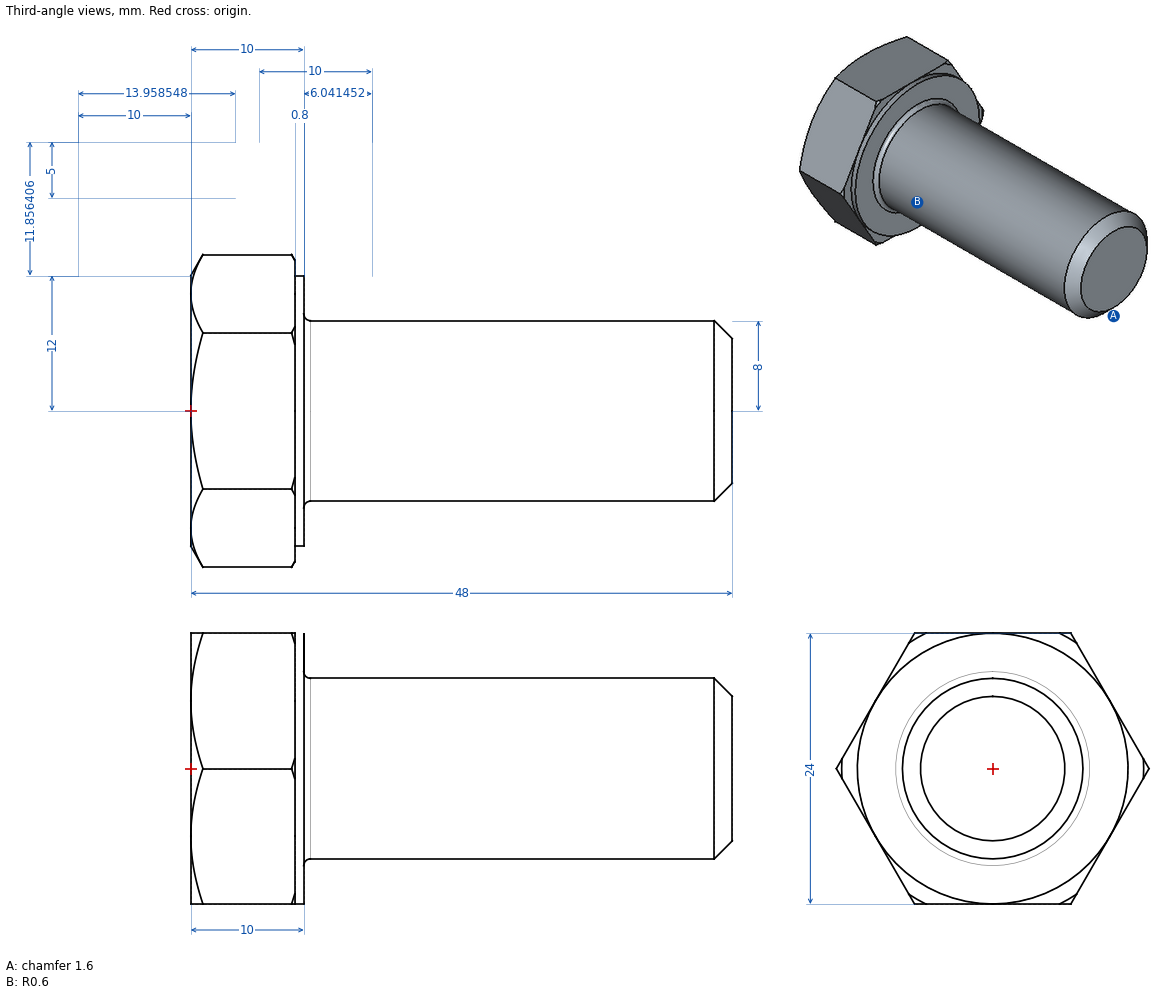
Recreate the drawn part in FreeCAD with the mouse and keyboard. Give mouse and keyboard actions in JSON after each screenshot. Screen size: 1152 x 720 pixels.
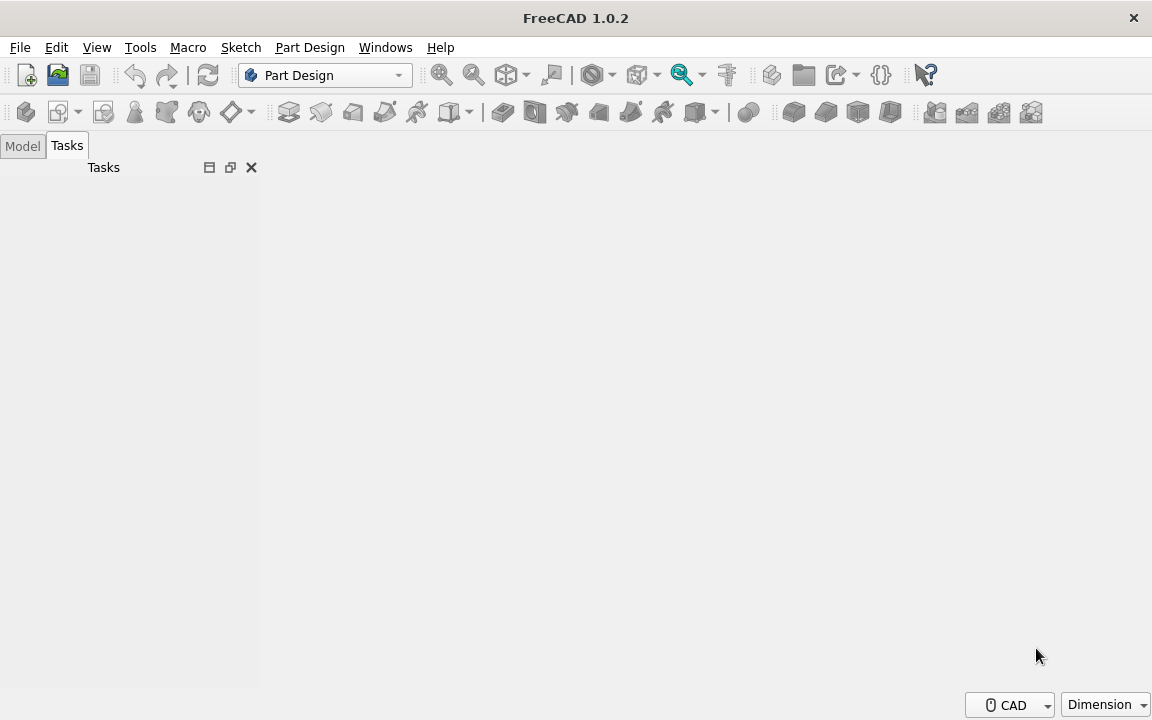
{"action": "left_click", "coordinate": [26, 76]}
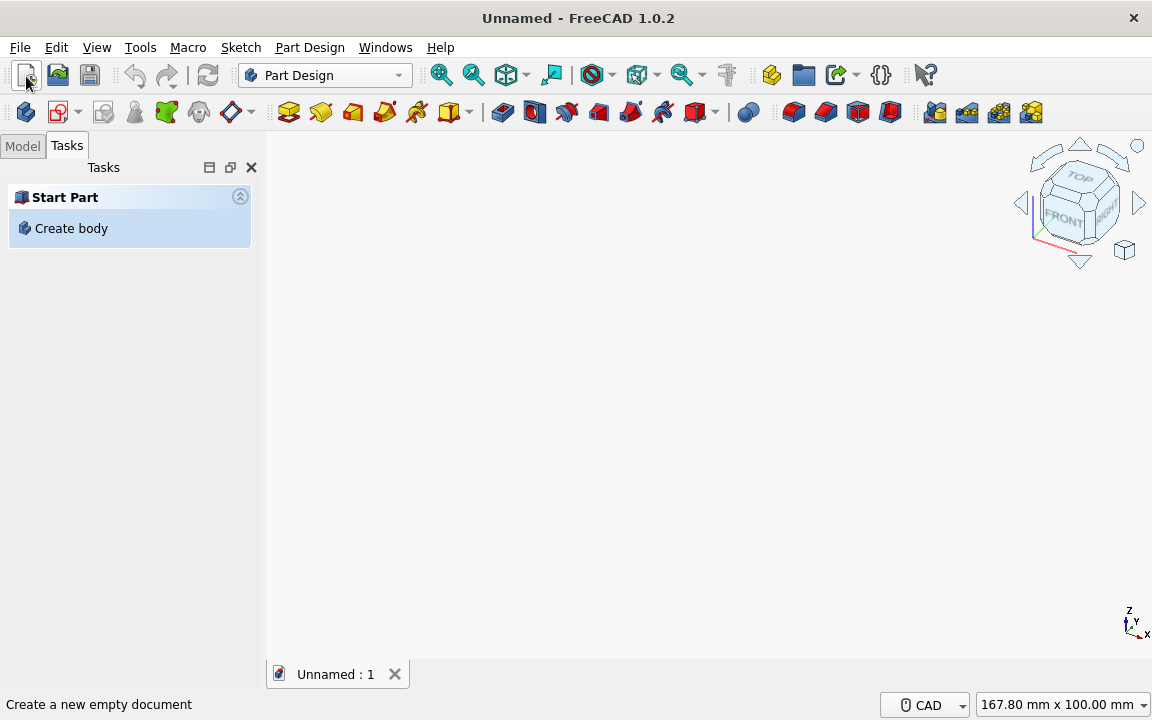
{"action": "left_click", "coordinate": [58, 112]}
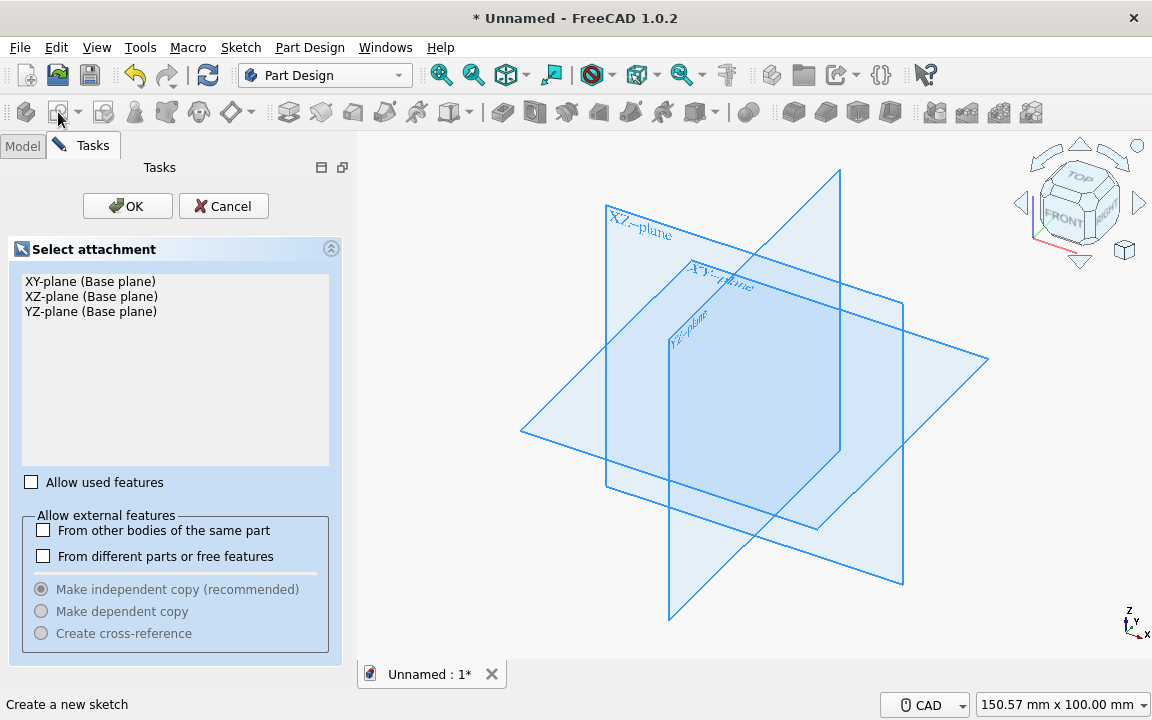
{"action": "left_click", "coordinate": [82, 312]}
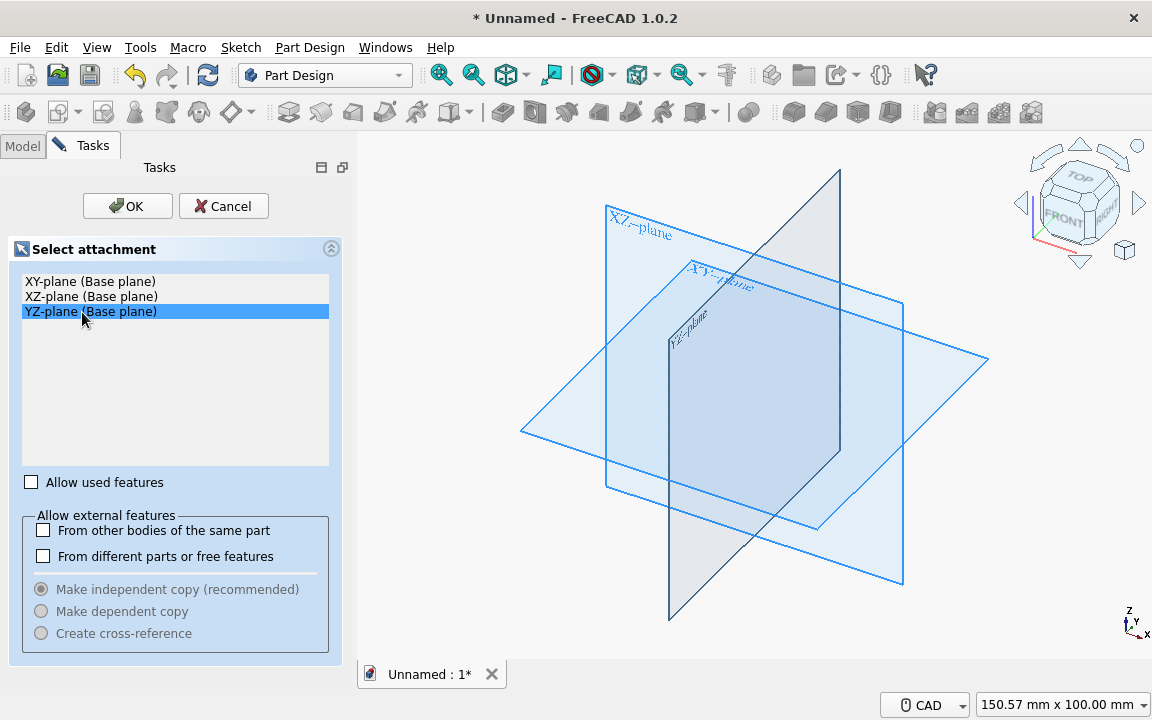
{"action": "left_click", "coordinate": [128, 206]}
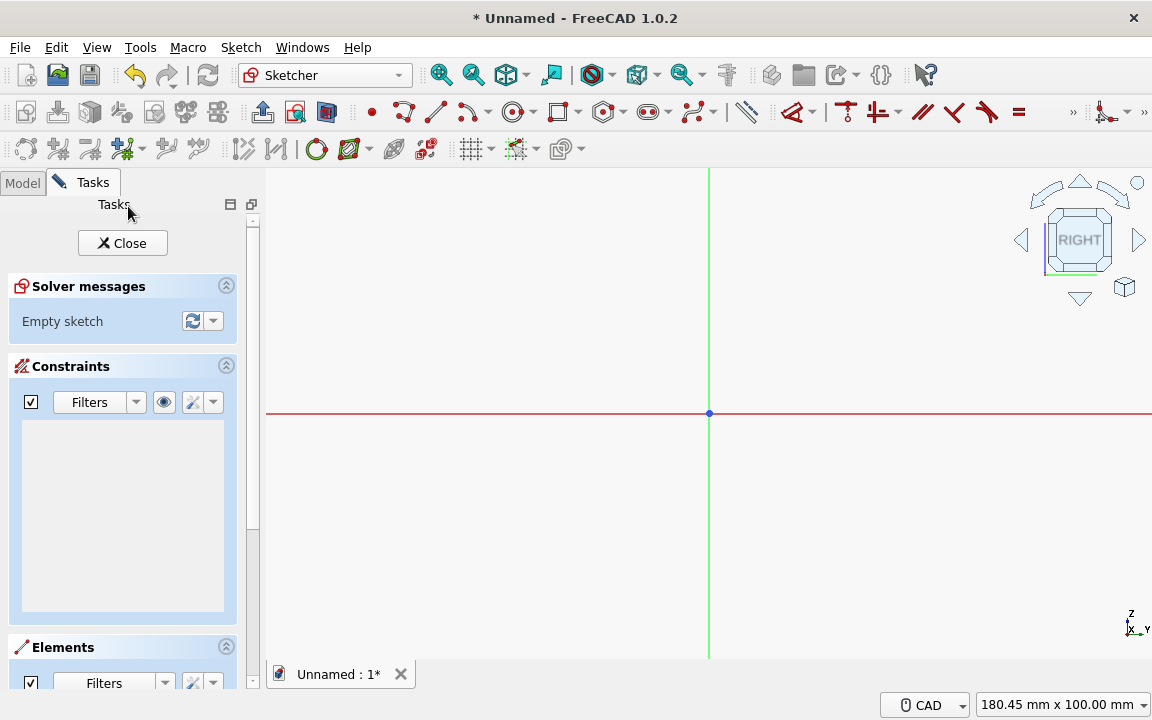
{"action": "scroll", "coordinate": [749, 414], "scroll_direction": "up", "scroll_amount": 5}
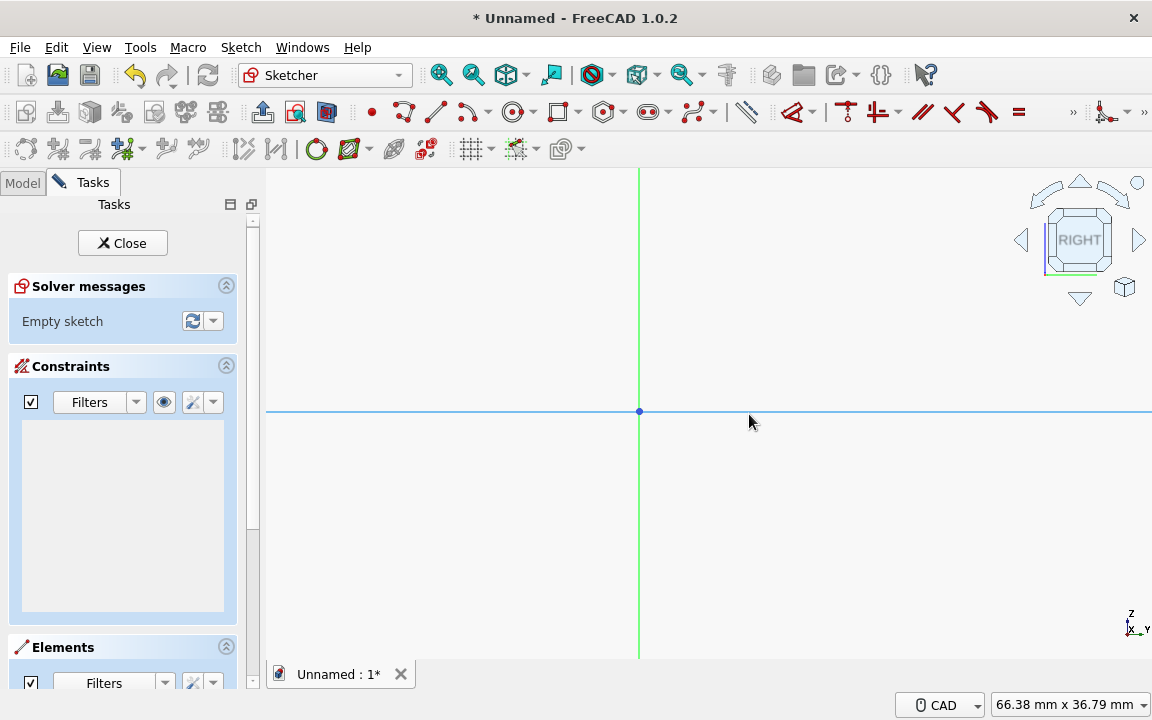
{"action": "left_click", "coordinate": [604, 112]}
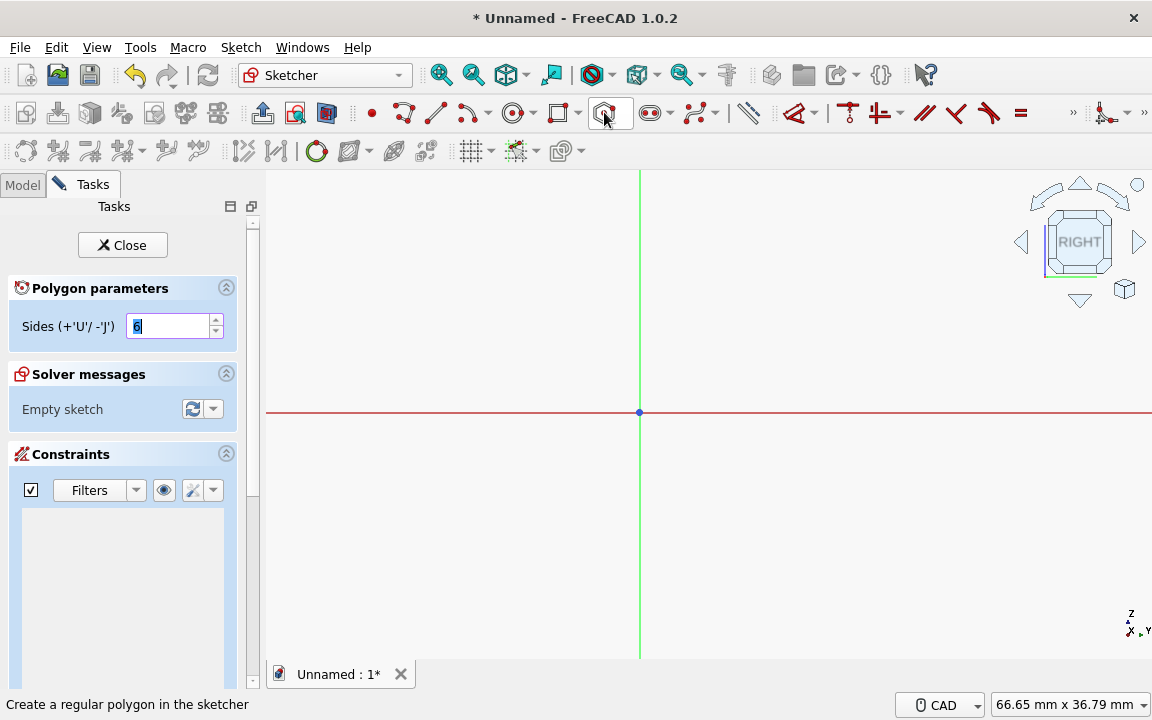
{"action": "left_click", "coordinate": [640, 413]}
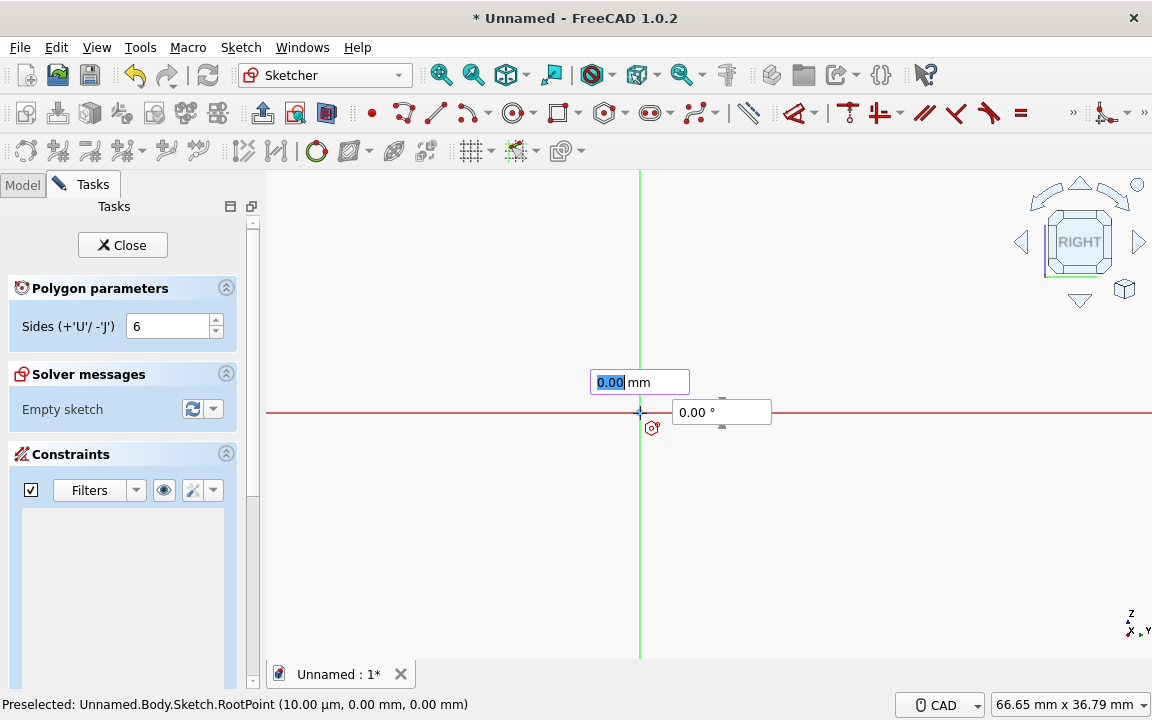
{"action": "left_click", "coordinate": [824, 413]}
{"action": "key", "text": "Escape"}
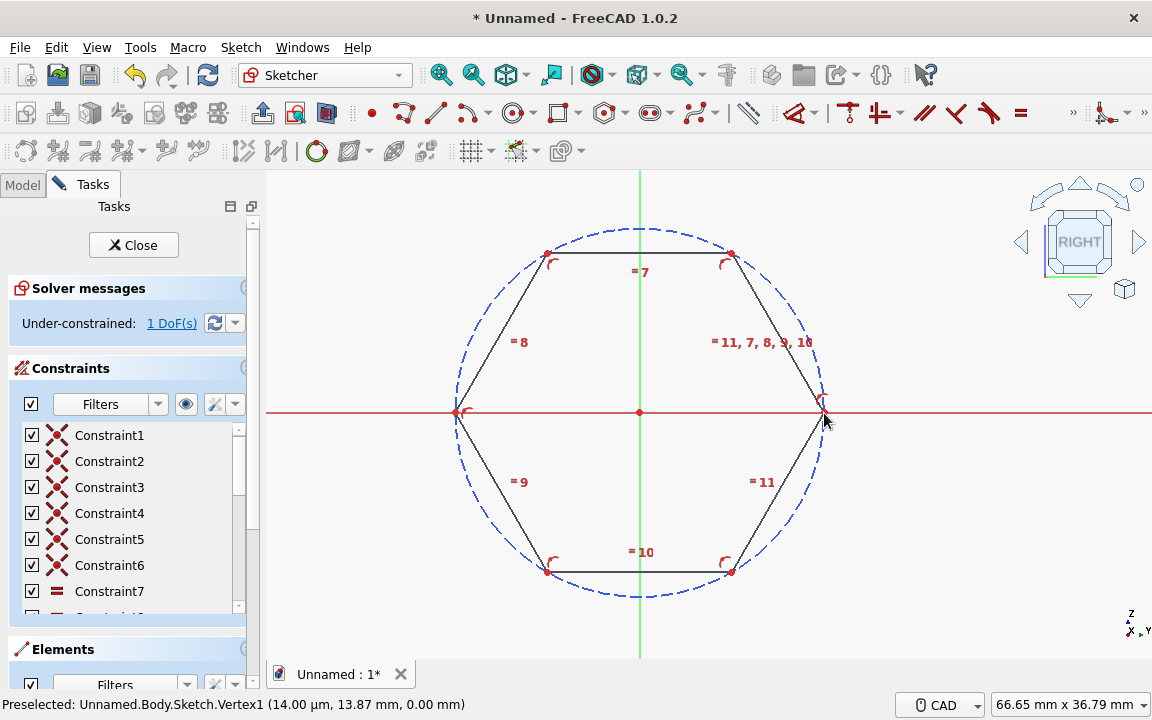
{"action": "left_click", "coordinate": [794, 114]}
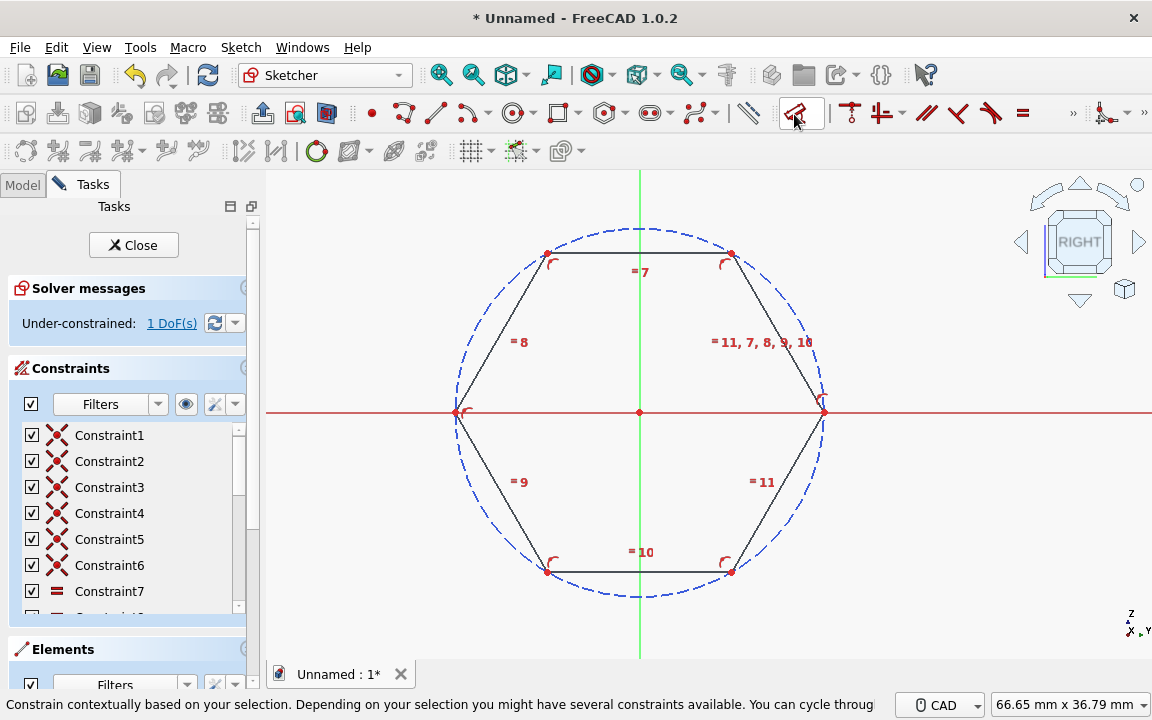
{"action": "left_click", "coordinate": [547, 572]}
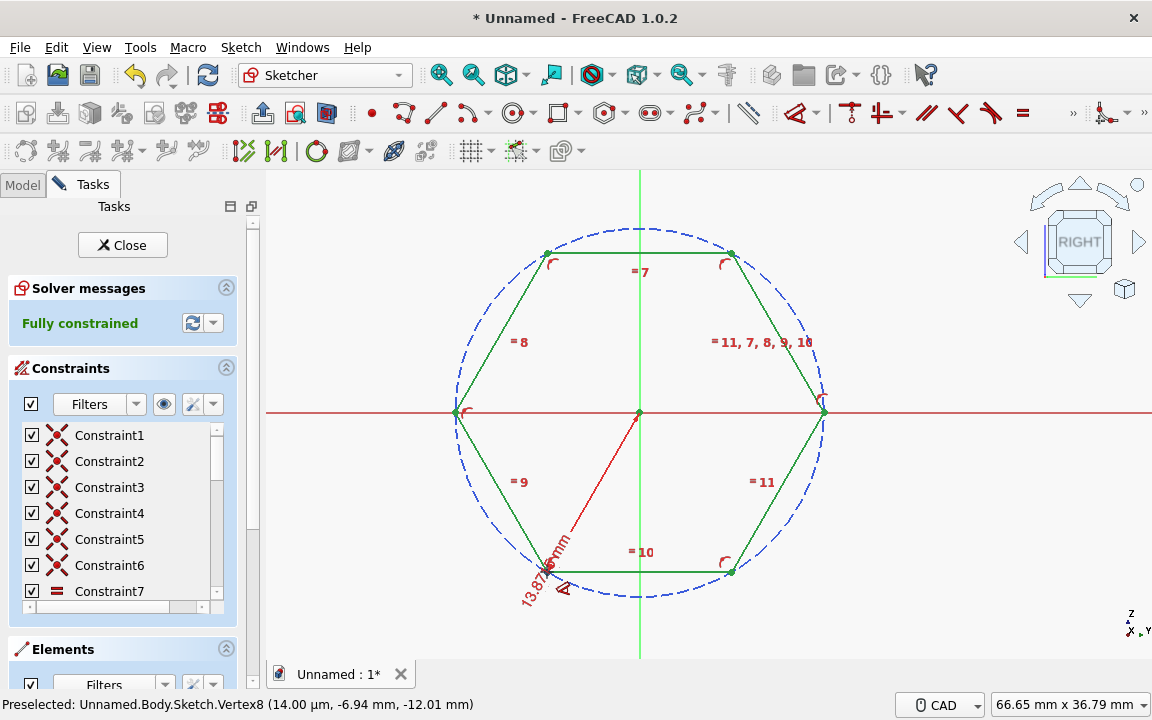
{"action": "left_click", "coordinate": [732, 253]}
{"action": "left_click", "coordinate": [766, 339]}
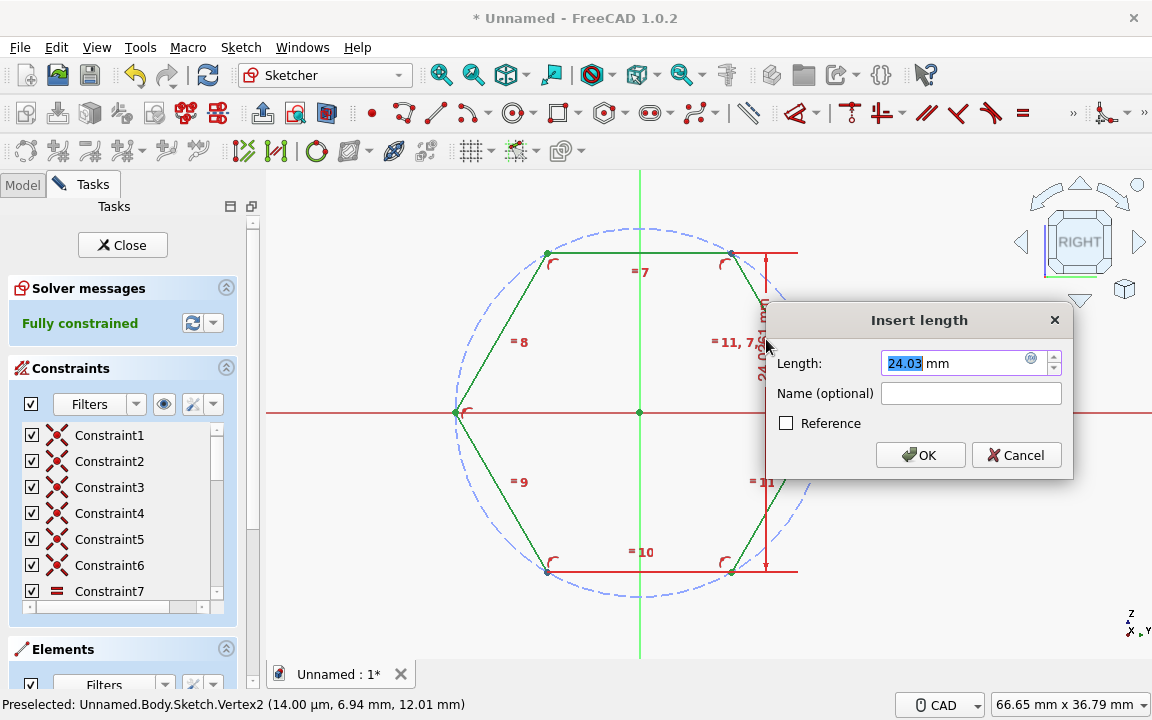
{"action": "type", "text": "24"}
{"action": "key", "text": "Return"}
{"action": "key", "text": "Escape"}